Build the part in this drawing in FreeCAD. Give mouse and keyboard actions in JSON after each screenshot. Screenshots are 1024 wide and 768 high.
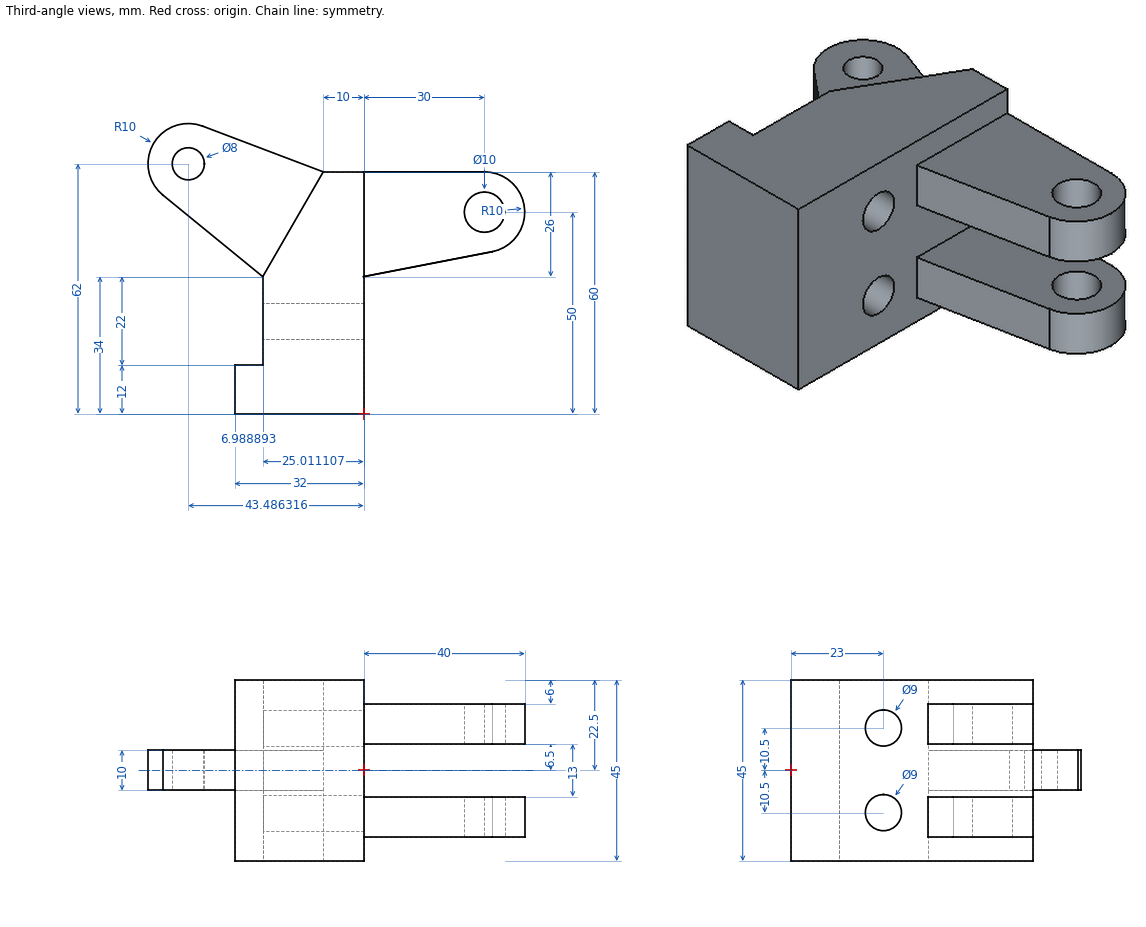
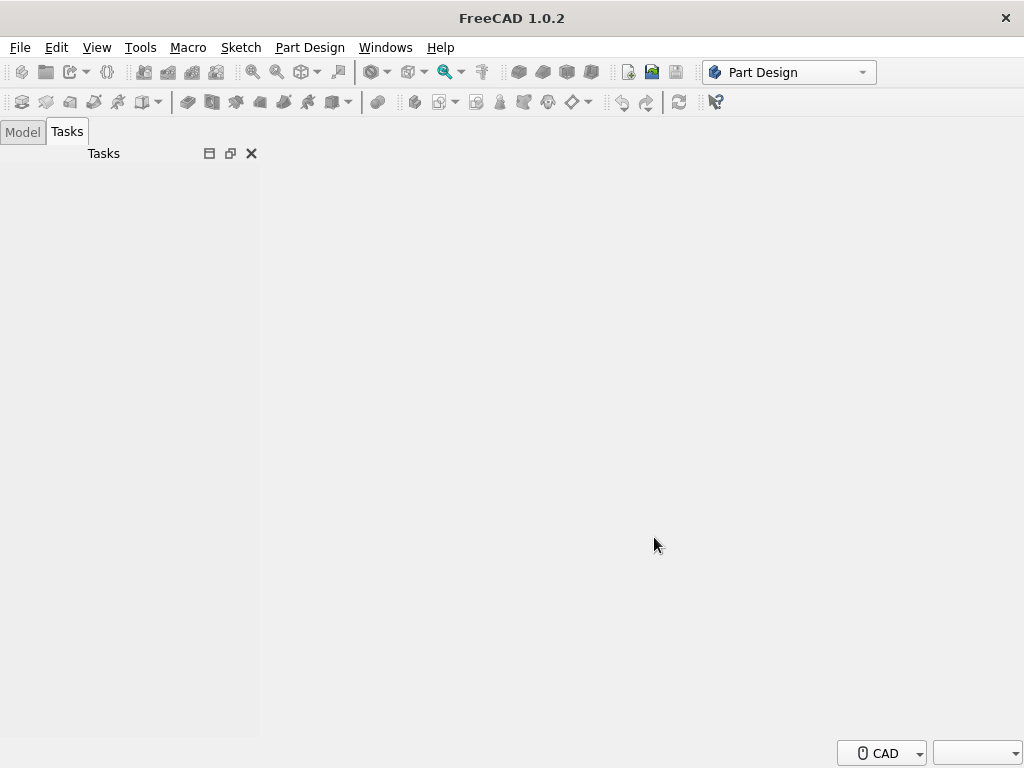
{"action": "left_click", "coordinate": [628, 72]}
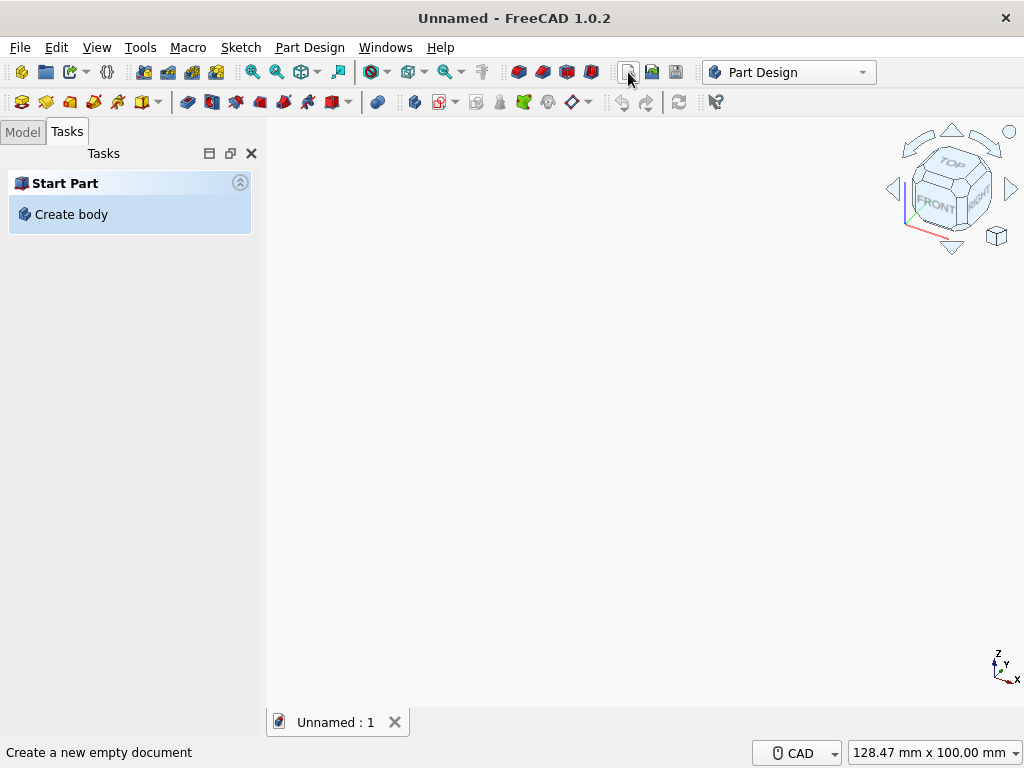
{"action": "left_click", "coordinate": [440, 102]}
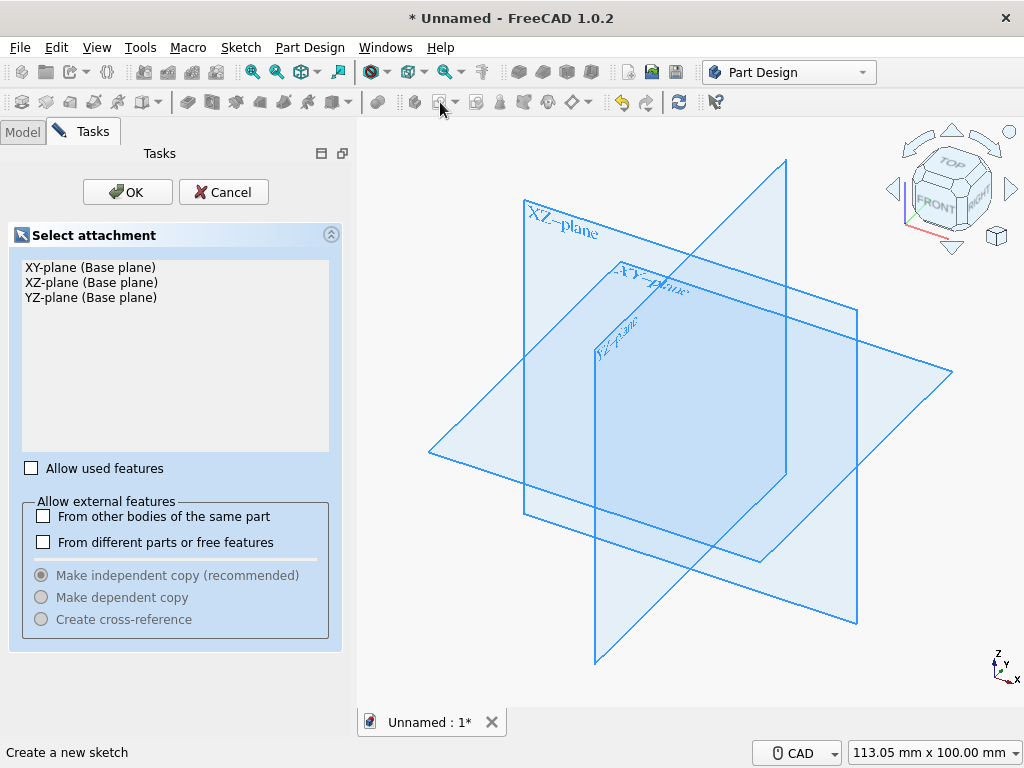
{"action": "left_click", "coordinate": [82, 268]}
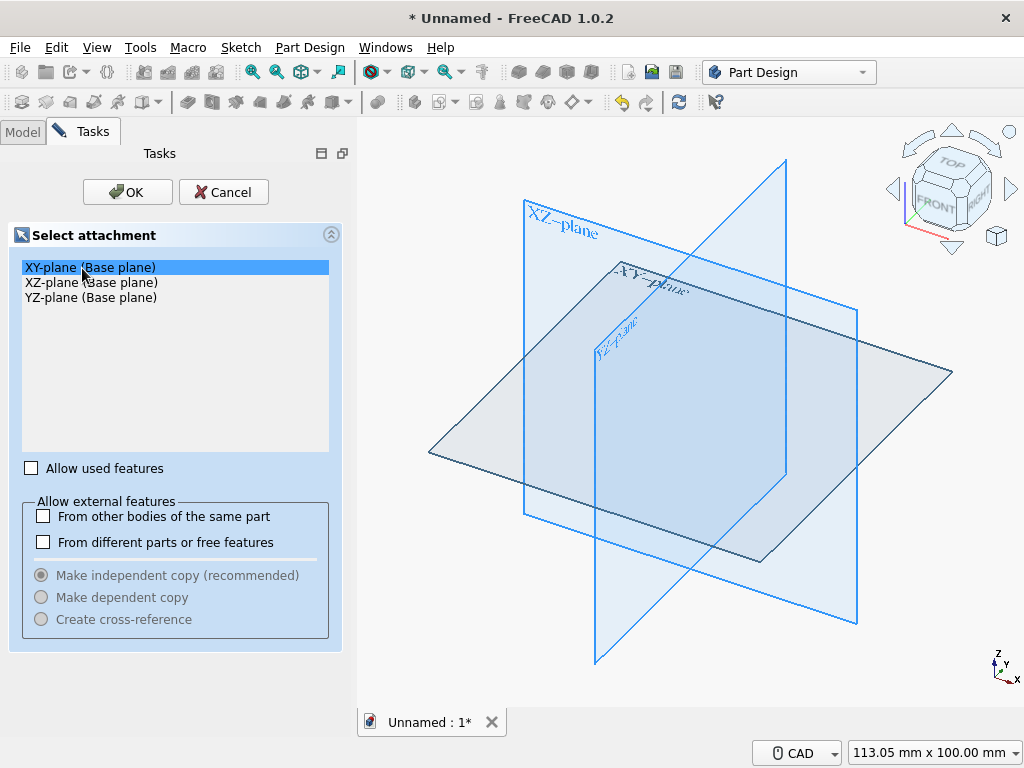
{"action": "left_click", "coordinate": [128, 192]}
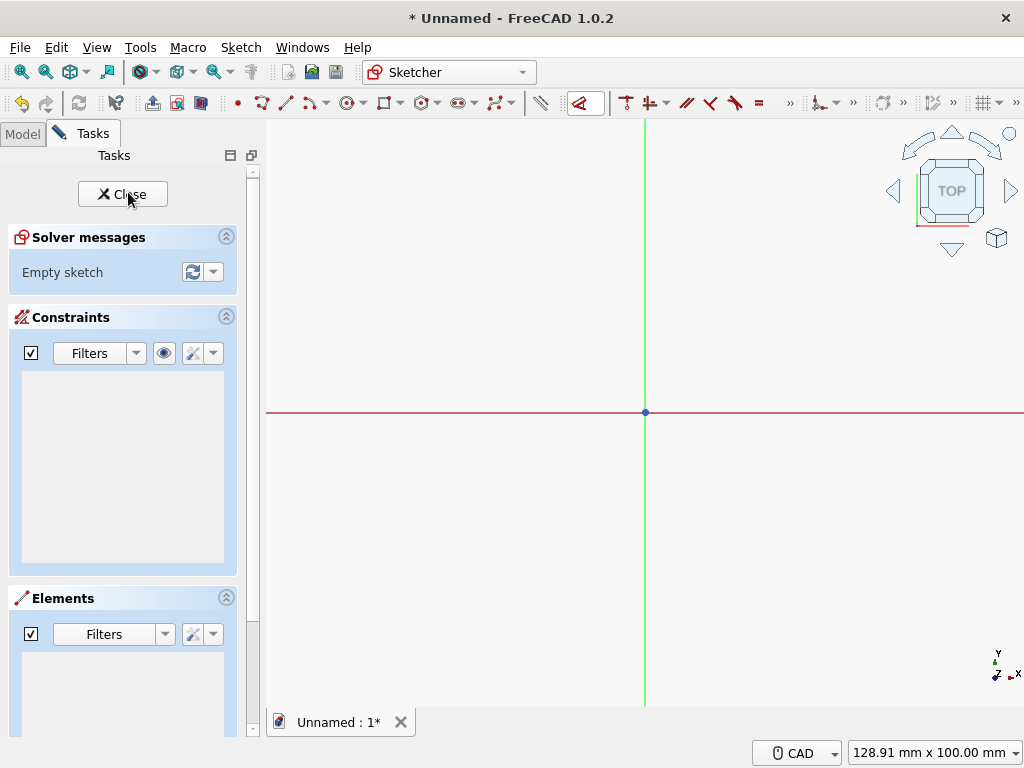
{"action": "scroll", "coordinate": [692, 679], "scroll_direction": "down", "scroll_amount": 1}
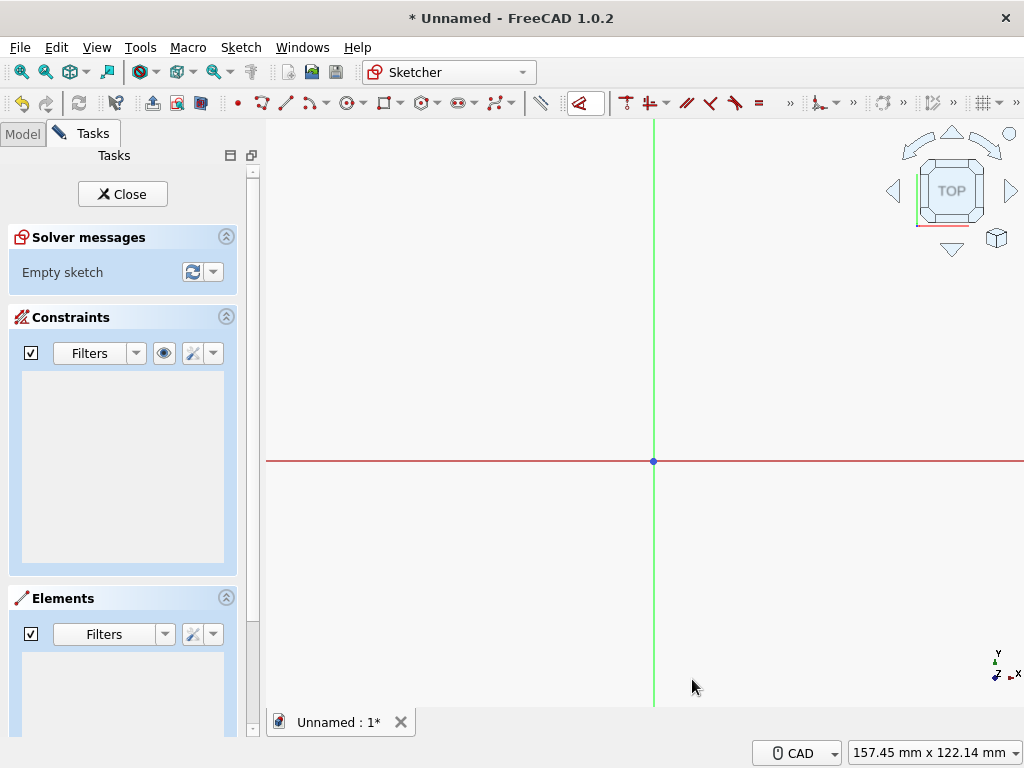
{"action": "key", "text": "g m"}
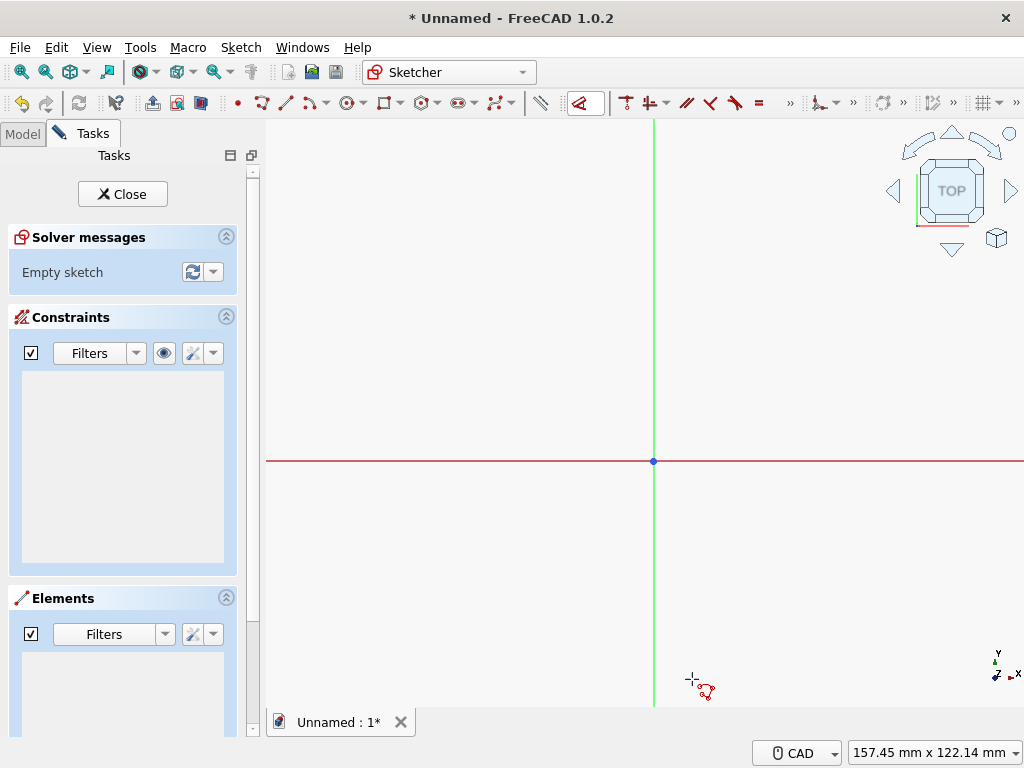
{"action": "left_click", "coordinate": [654, 461]}
{"action": "left_click", "coordinate": [645, 173]}
{"action": "left_click", "coordinate": [605, 173]}
{"action": "left_click", "coordinate": [533, 298]}
{"action": "left_click", "coordinate": [533, 404]}
{"action": "left_click", "coordinate": [500, 404]}
{"action": "left_click", "coordinate": [500, 452]}
{"action": "left_click", "coordinate": [654, 461]}
{"action": "key", "text": "Escape"}
{"action": "key", "text": "Escape"}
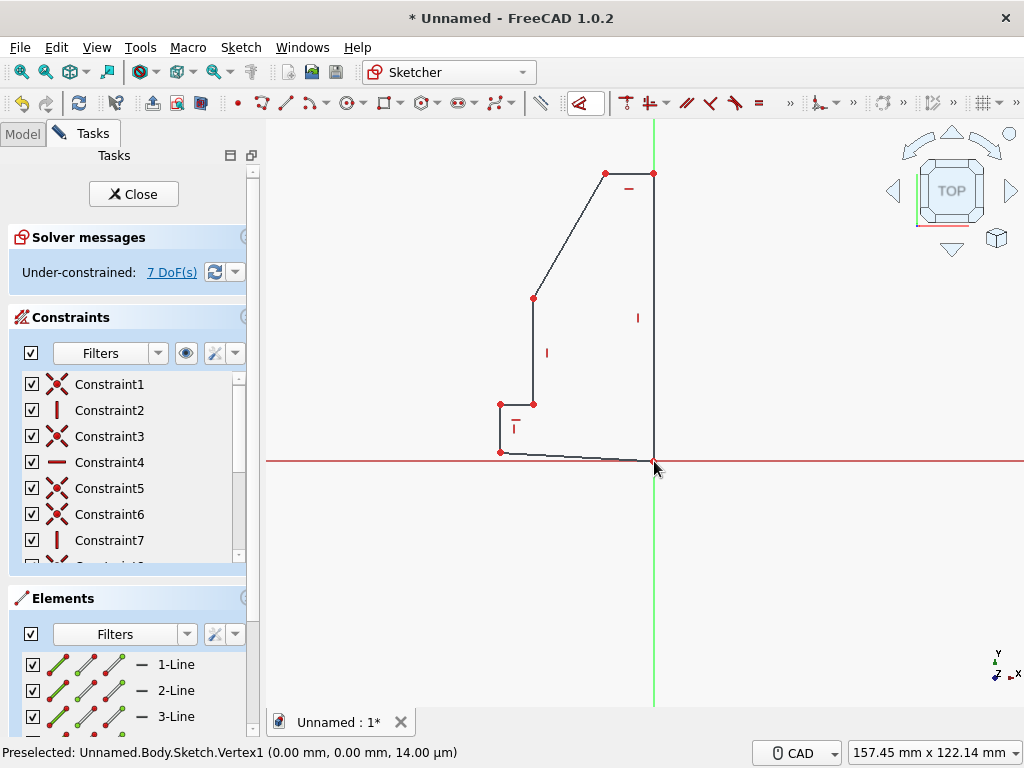
{"action": "left_click", "coordinate": [608, 459]}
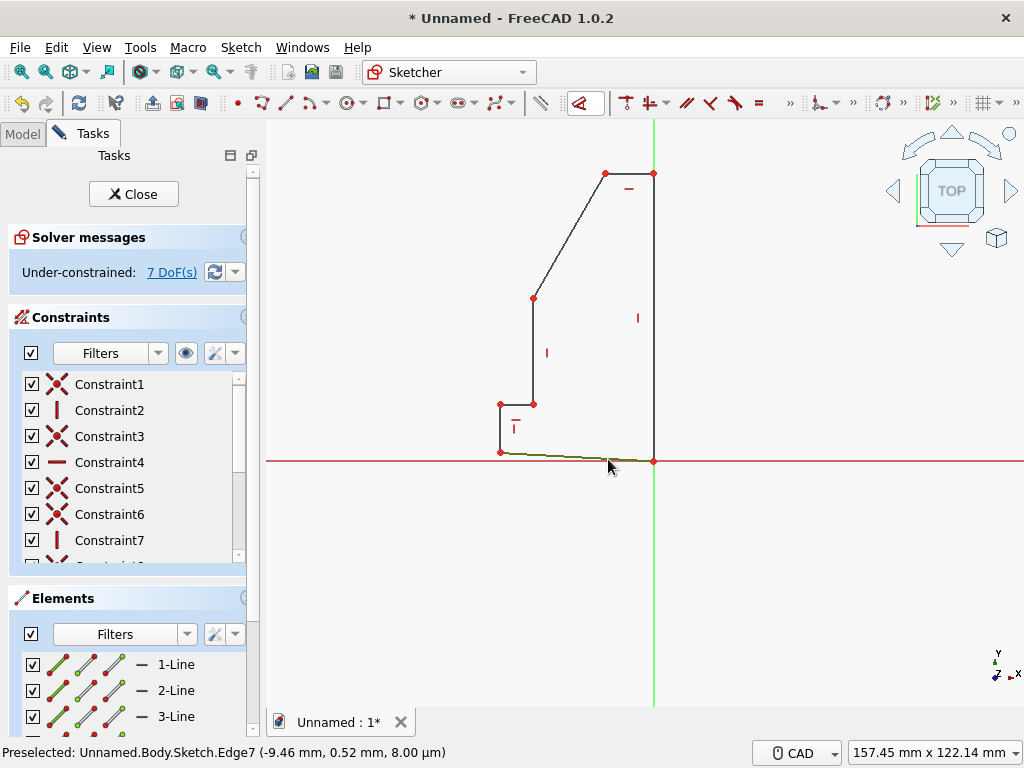
{"action": "key", "text": "h"}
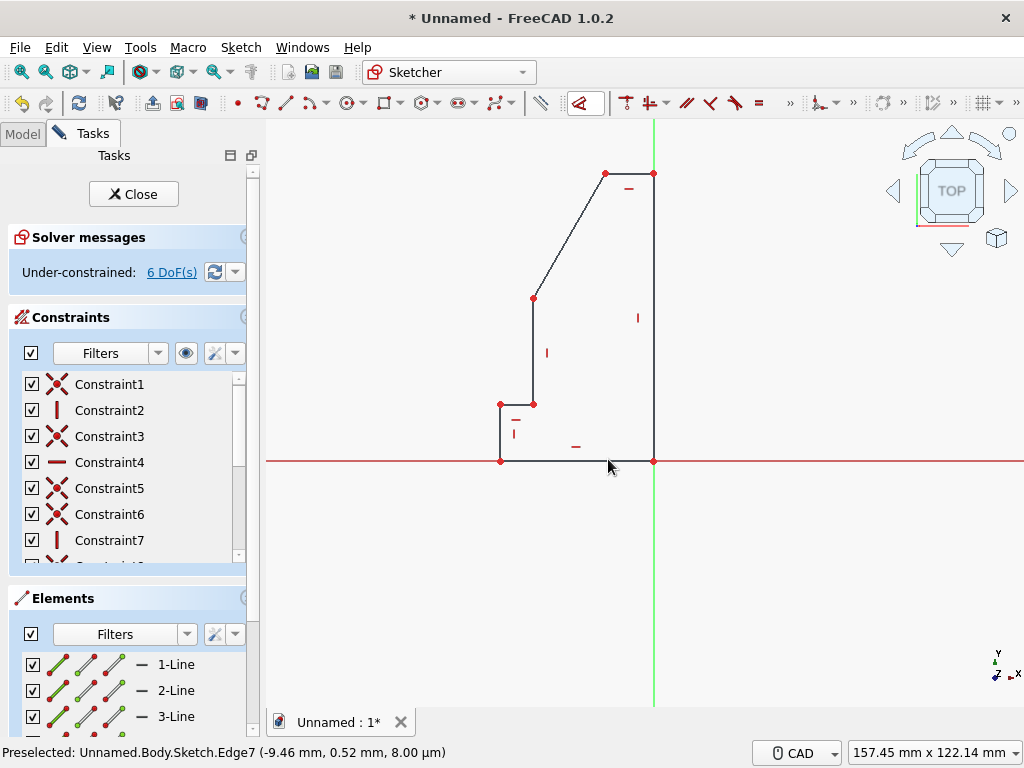
{"action": "left_click", "coordinate": [654, 375]}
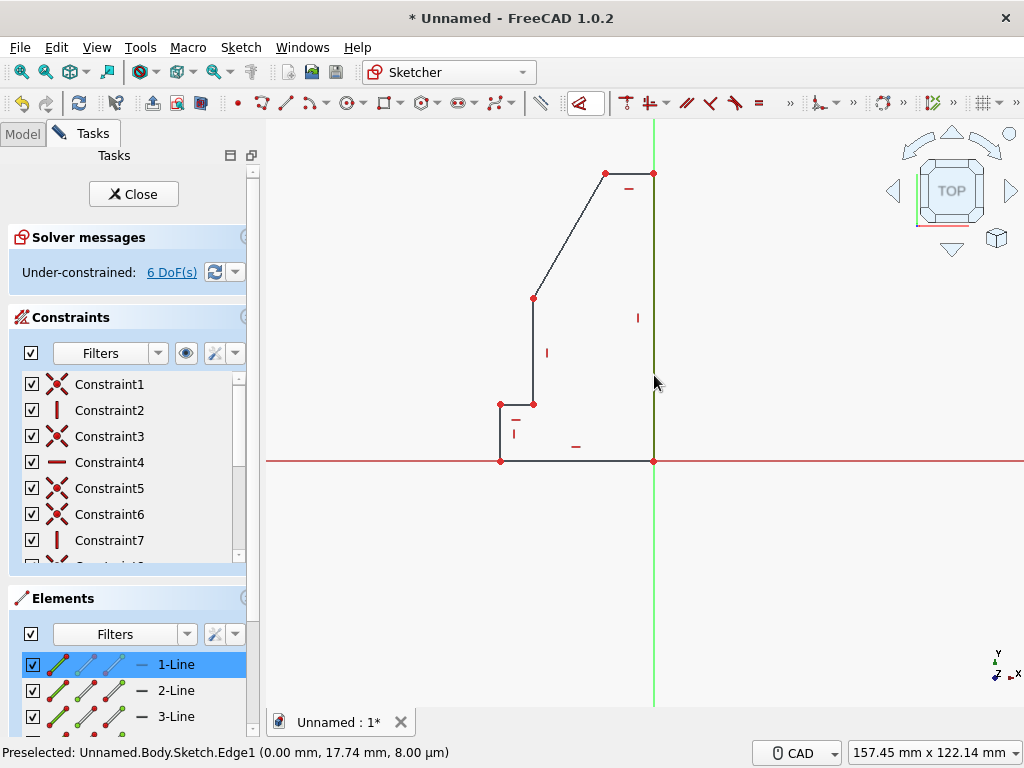
{"action": "key", "text": "i"}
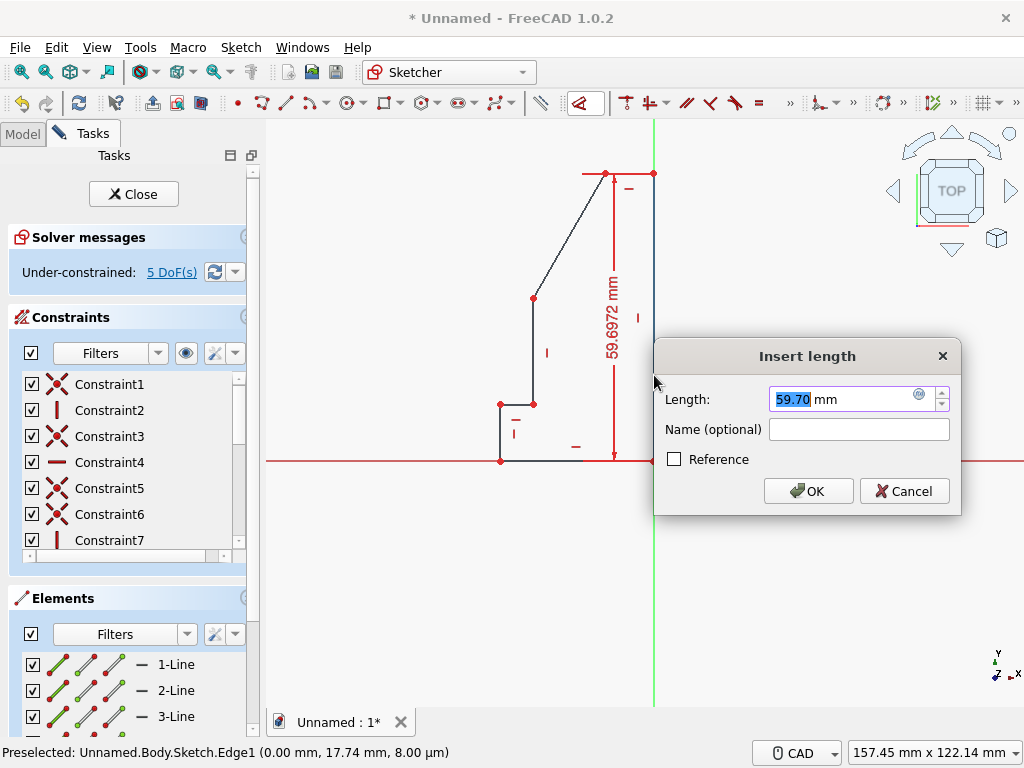
{"action": "type", "text": "60"}
{"action": "key", "text": "Return"}